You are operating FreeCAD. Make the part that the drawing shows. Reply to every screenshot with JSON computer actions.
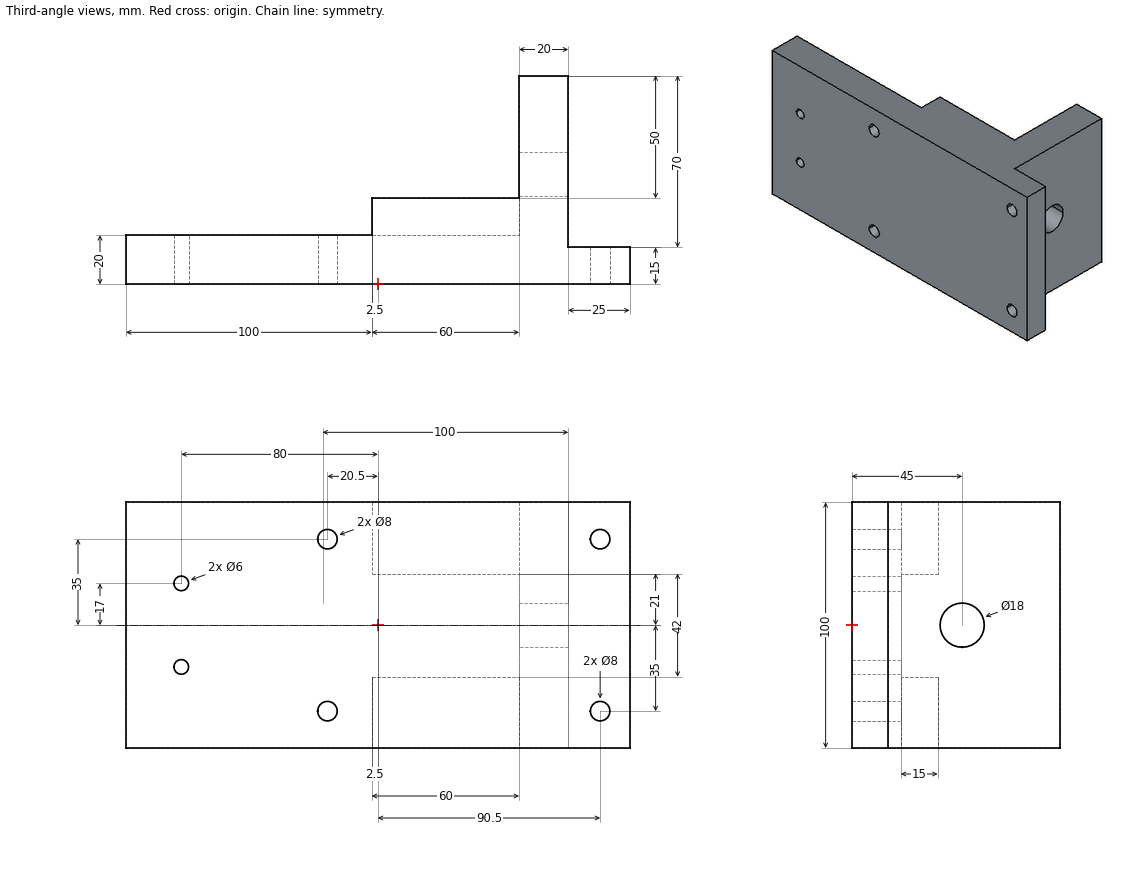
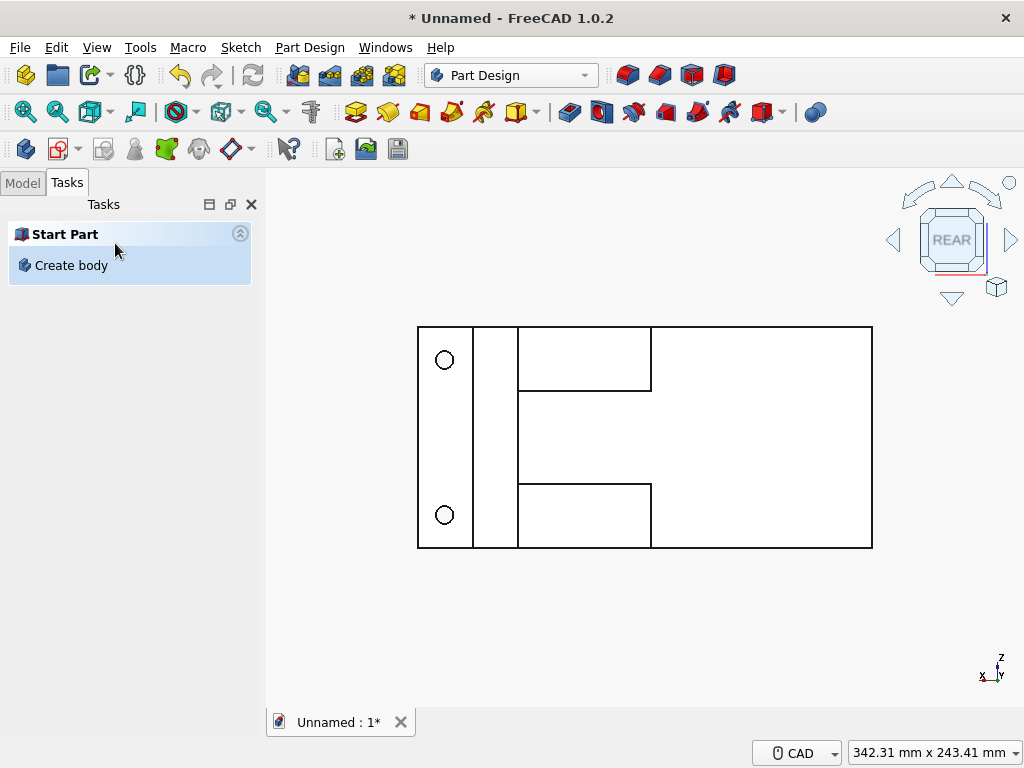
{"action": "left_click", "coordinate": [745, 437]}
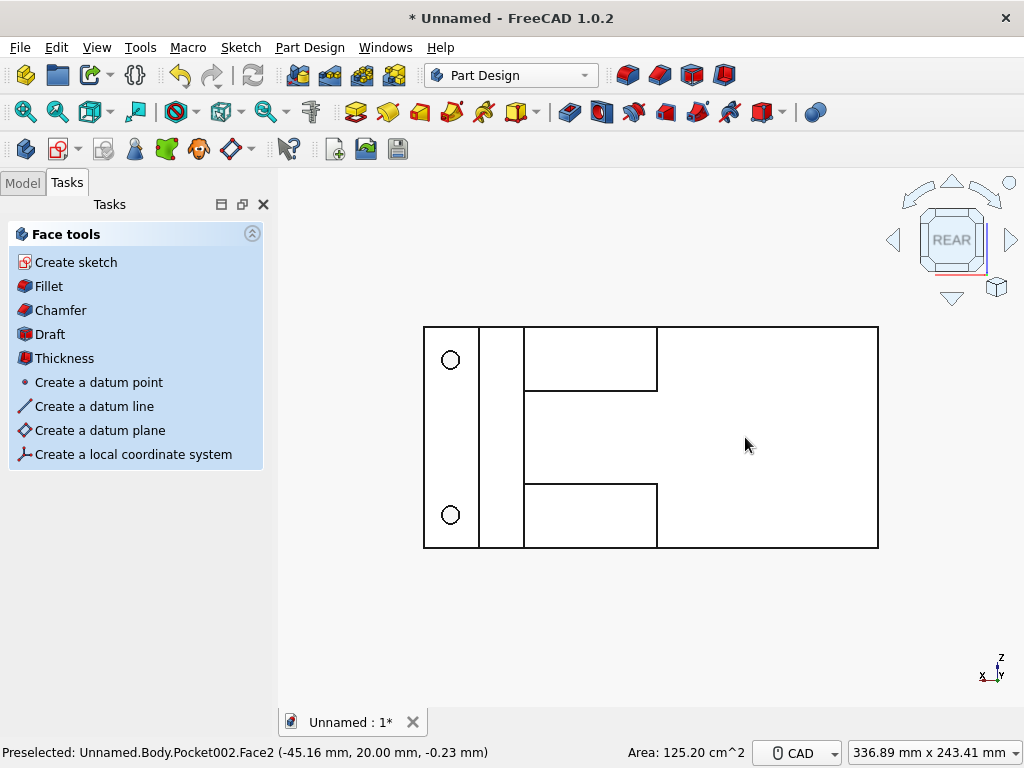
{"action": "left_click", "coordinate": [58, 150]}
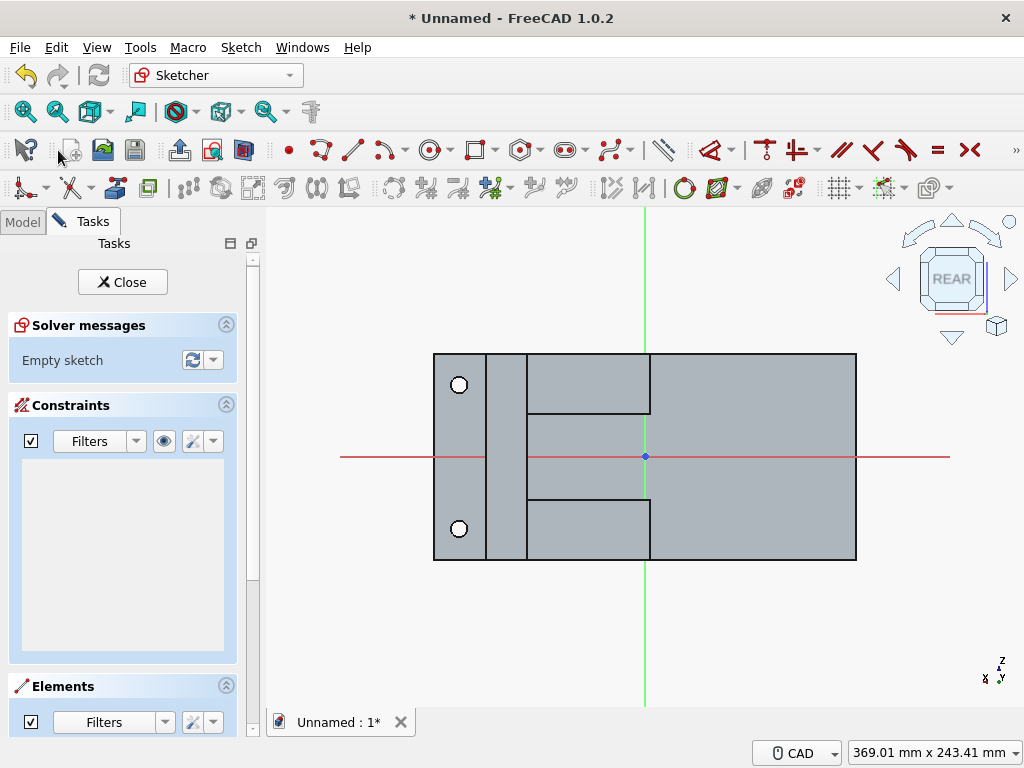
{"action": "scroll", "coordinate": [784, 457], "scroll_direction": "up", "scroll_amount": 3}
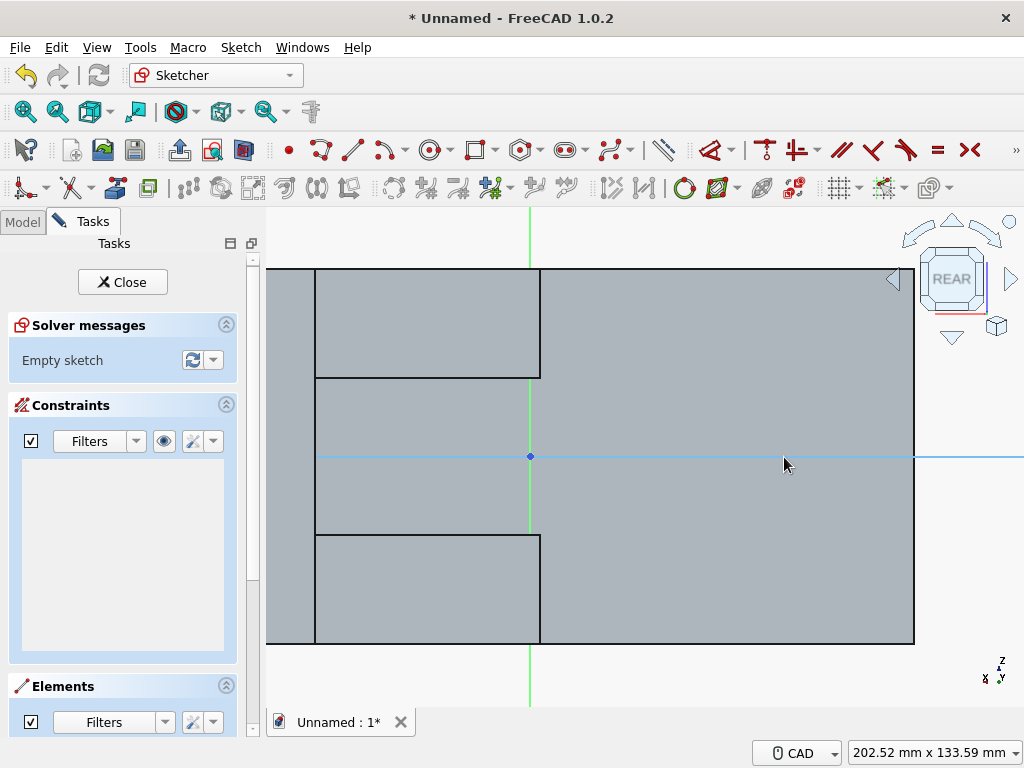
{"action": "left_click", "coordinate": [430, 150]}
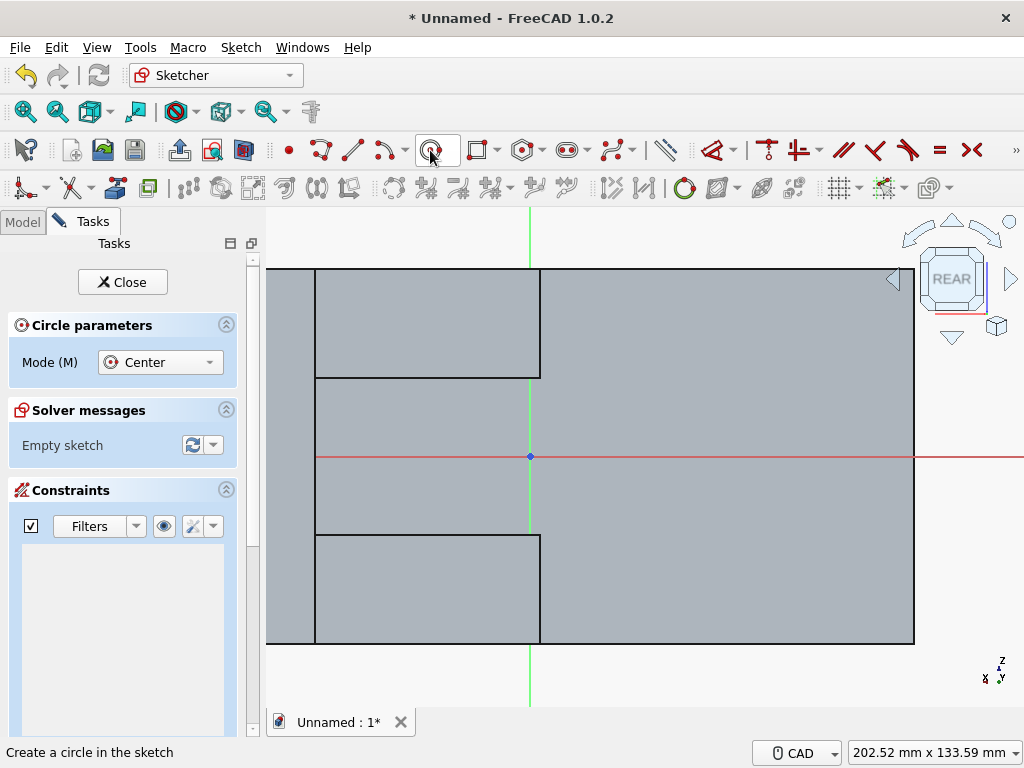
{"action": "scroll", "coordinate": [607, 326], "scroll_direction": "up", "scroll_amount": 3}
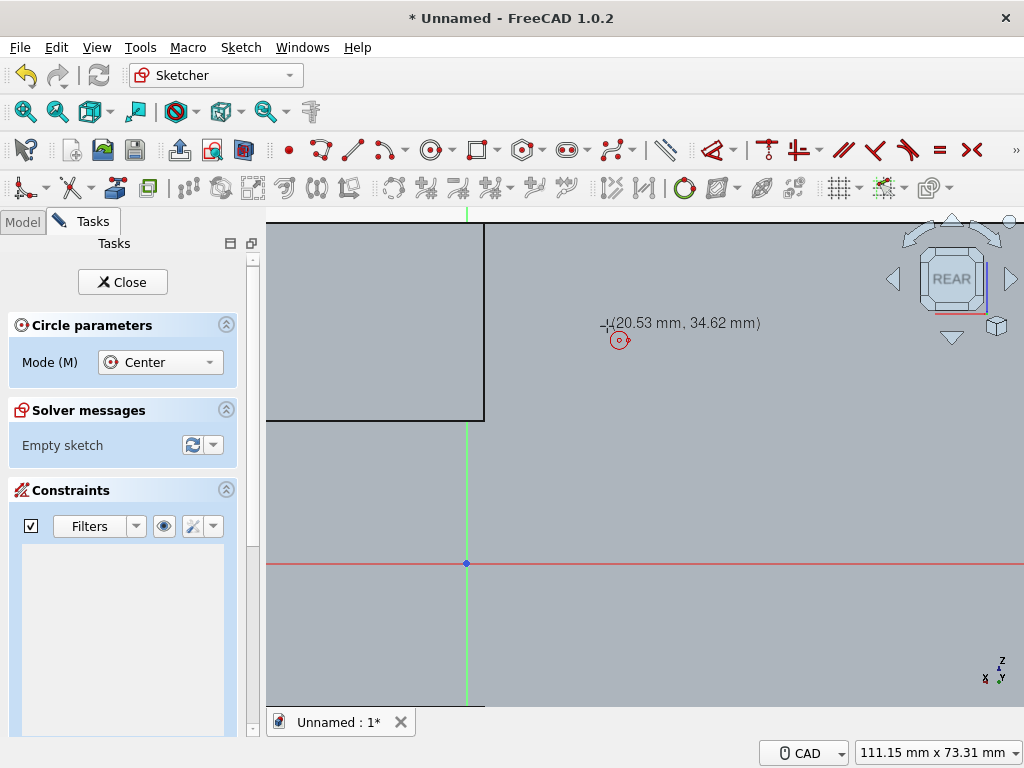
{"action": "left_click", "coordinate": [606, 325]}
{"action": "left_click", "coordinate": [626, 306]}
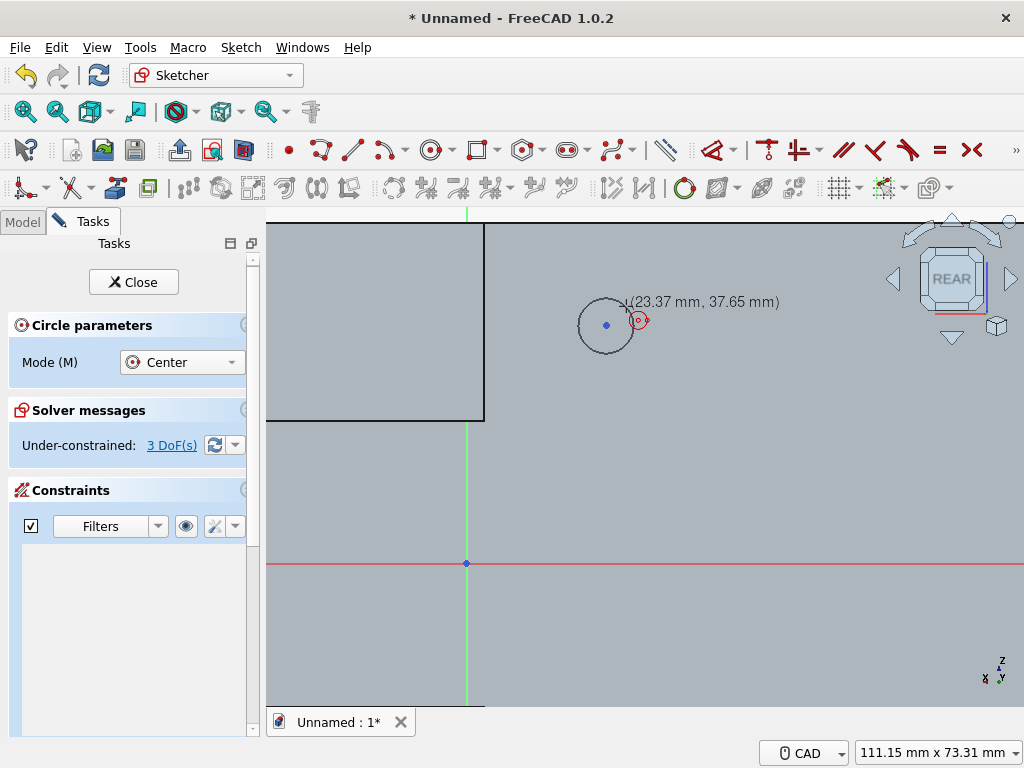
{"action": "scroll", "coordinate": [609, 327], "scroll_direction": "down", "scroll_amount": 3}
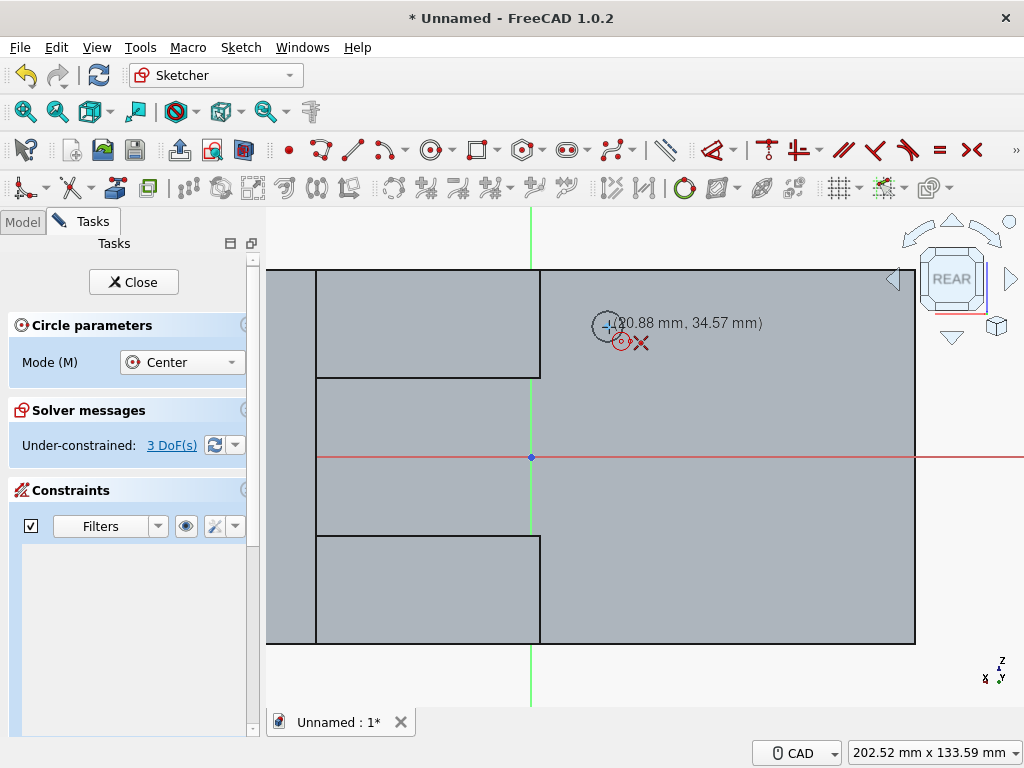
{"action": "scroll", "coordinate": [608, 588], "scroll_direction": "up", "scroll_amount": 3}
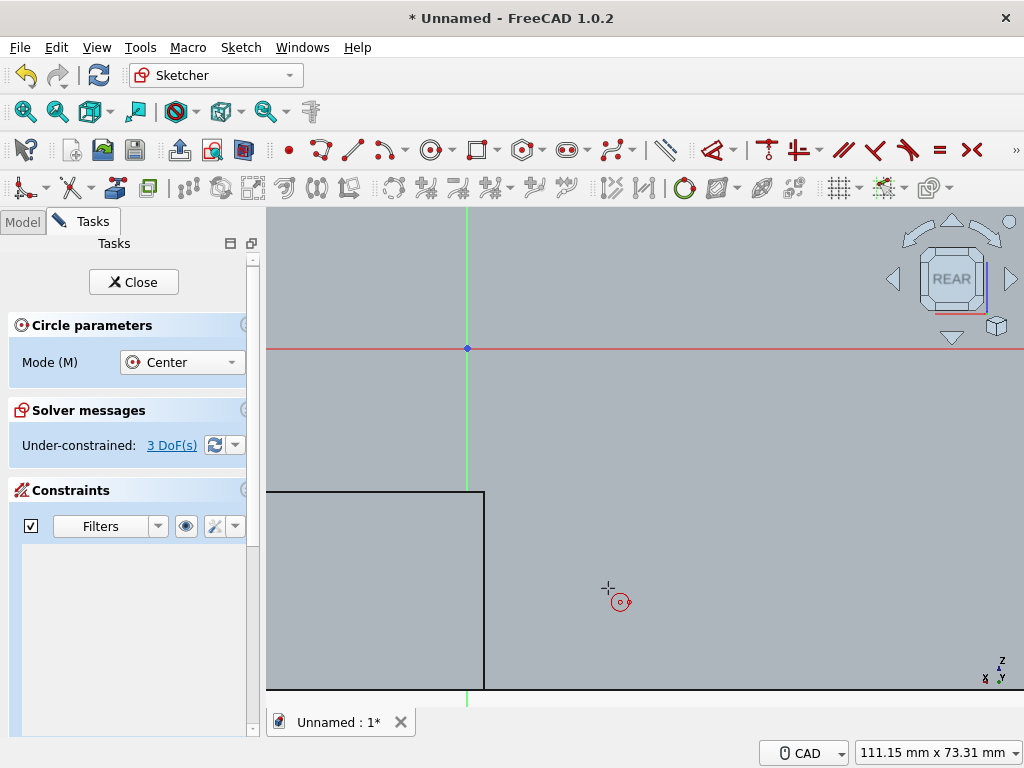
{"action": "left_click", "coordinate": [607, 587]}
{"action": "left_click", "coordinate": [627, 568]}
{"action": "key", "text": "Escape"}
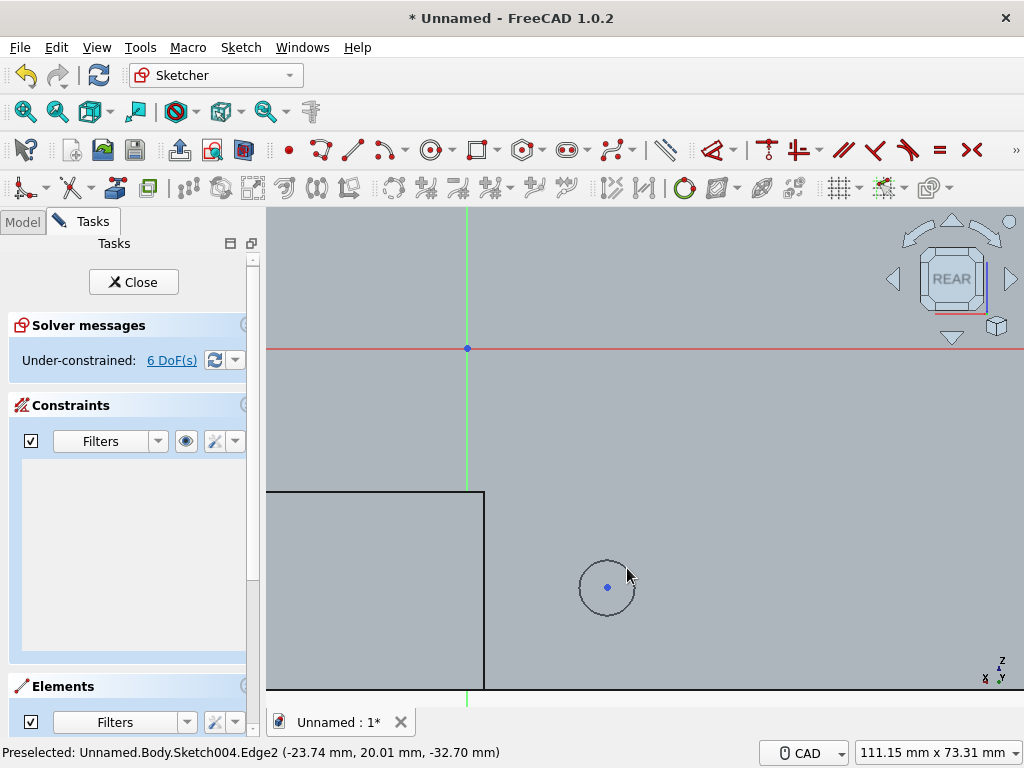
{"action": "scroll", "coordinate": [608, 589], "scroll_direction": "down", "scroll_amount": 3}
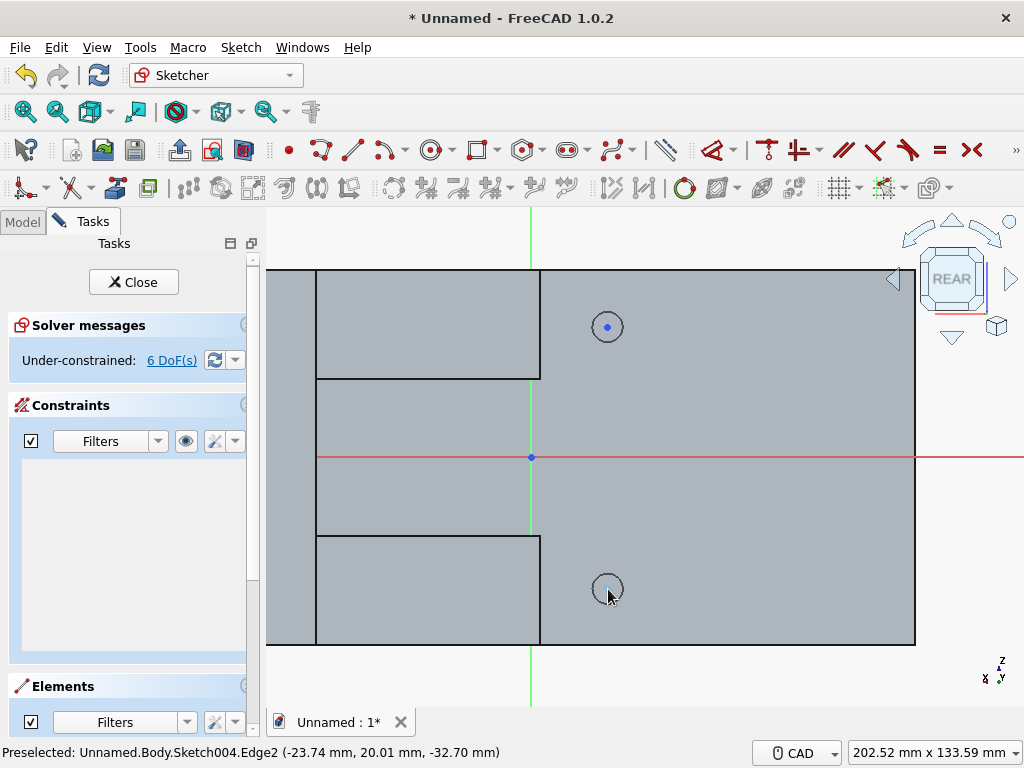
{"action": "left_click", "coordinate": [618, 316]}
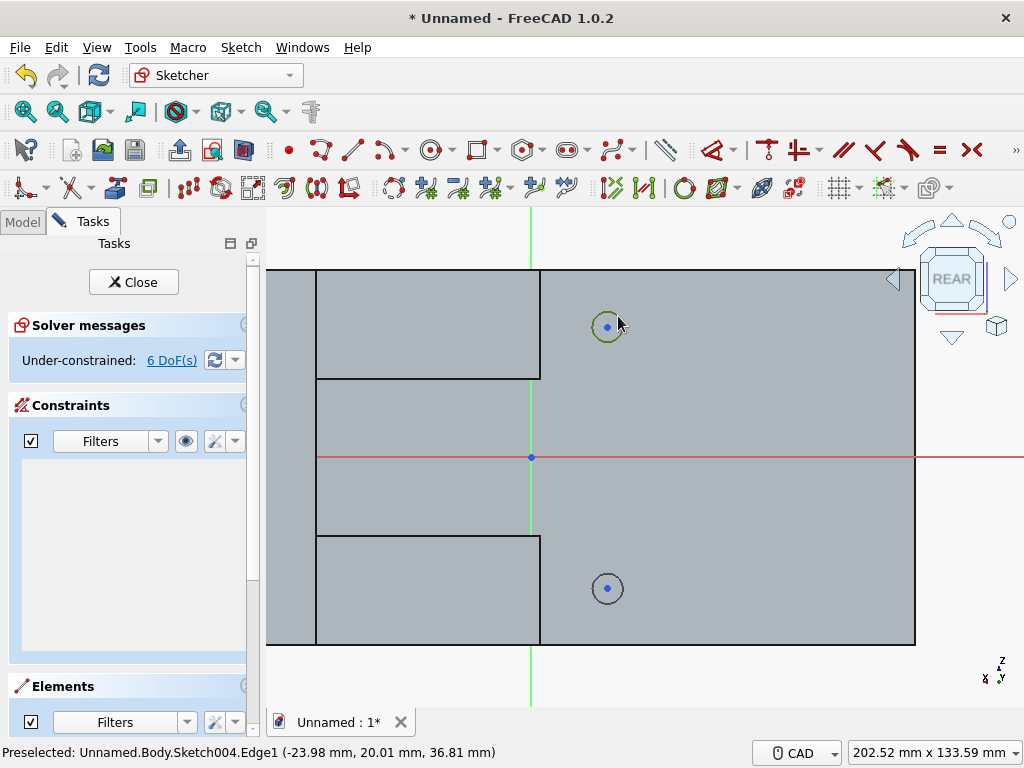
{"action": "left_click", "coordinate": [618, 578]}